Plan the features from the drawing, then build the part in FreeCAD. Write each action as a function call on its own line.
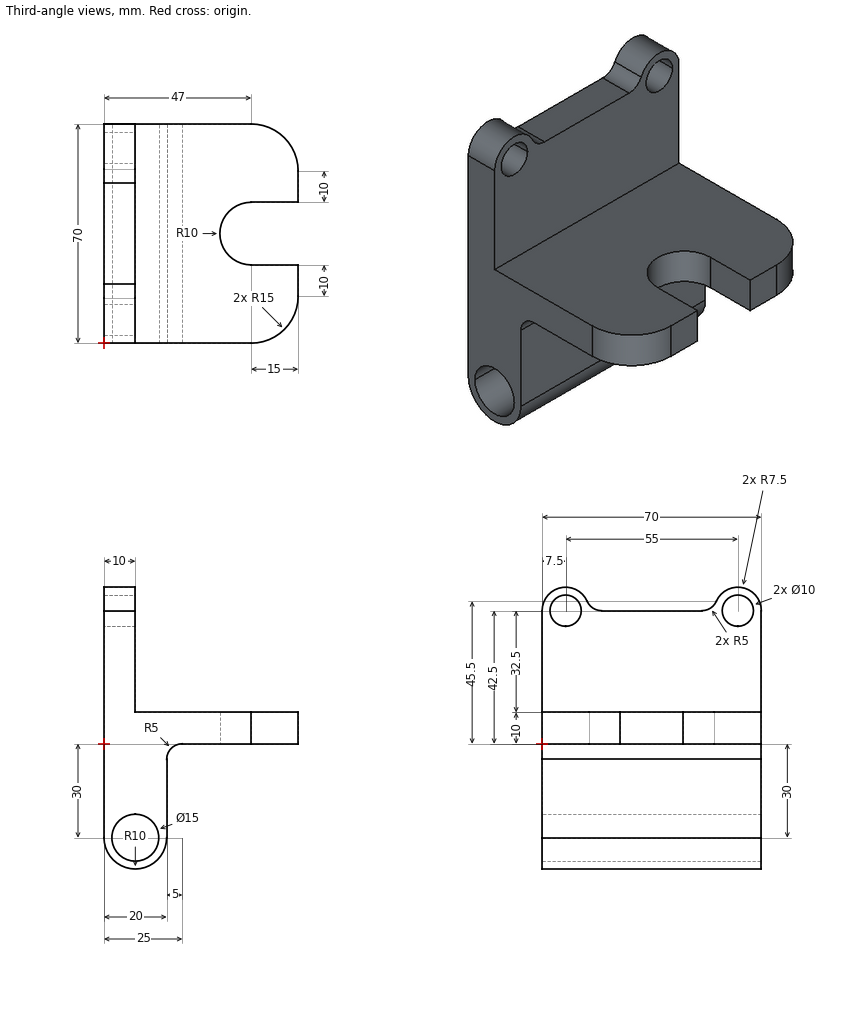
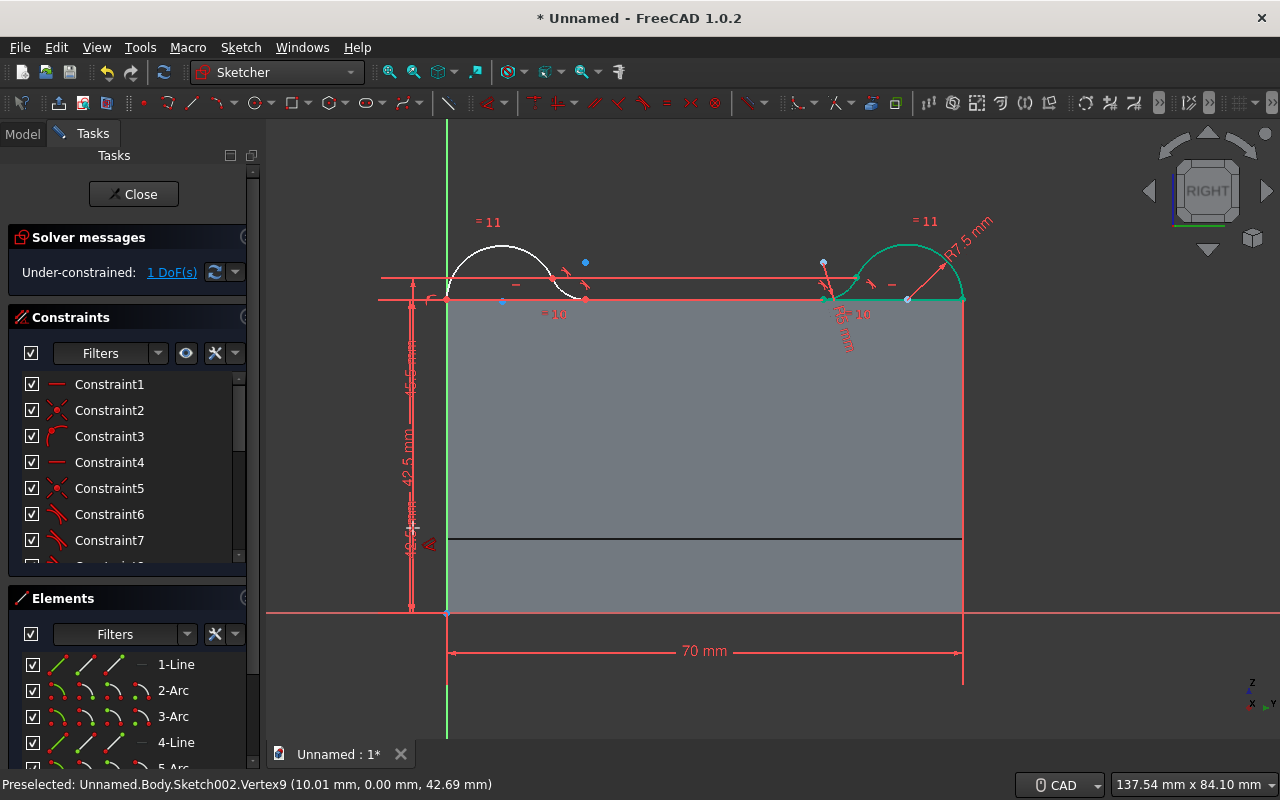
click(552, 278)
click(413, 329)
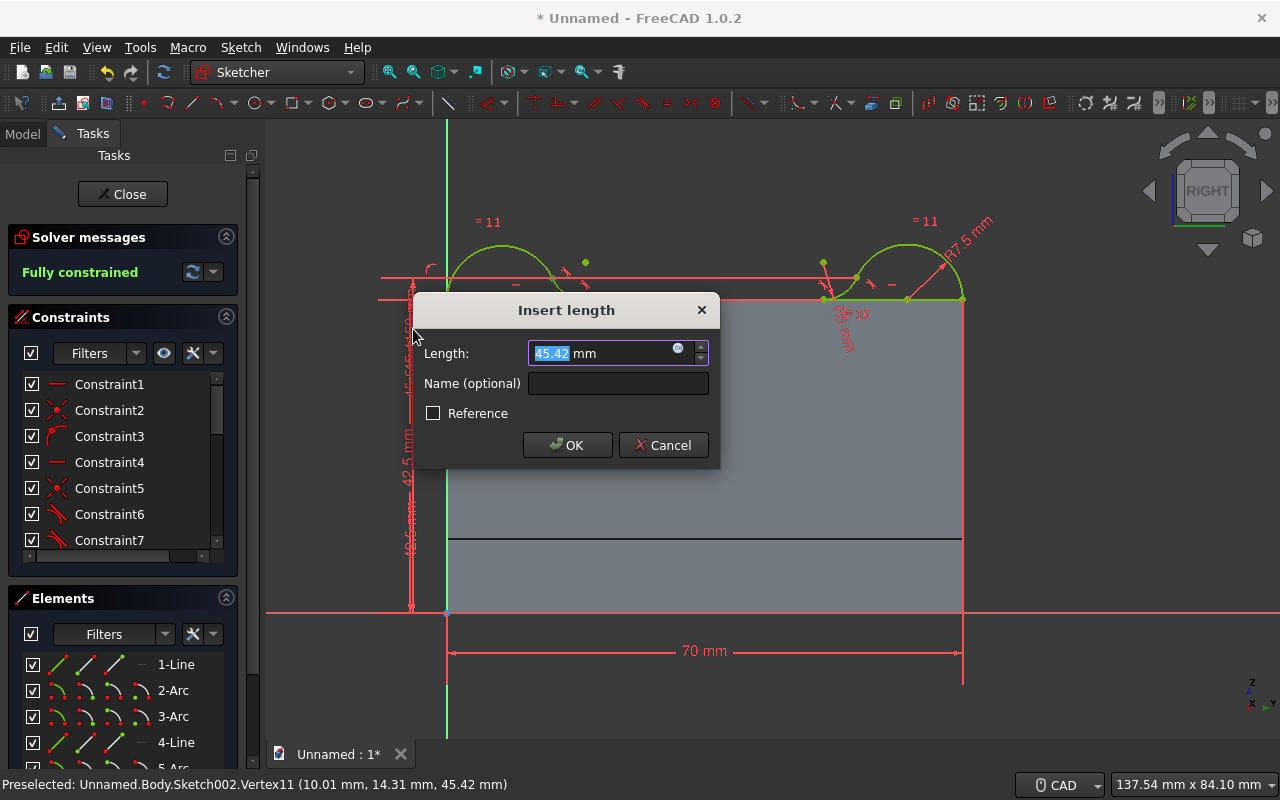
text(45.5)
key(Return)
key(Escape)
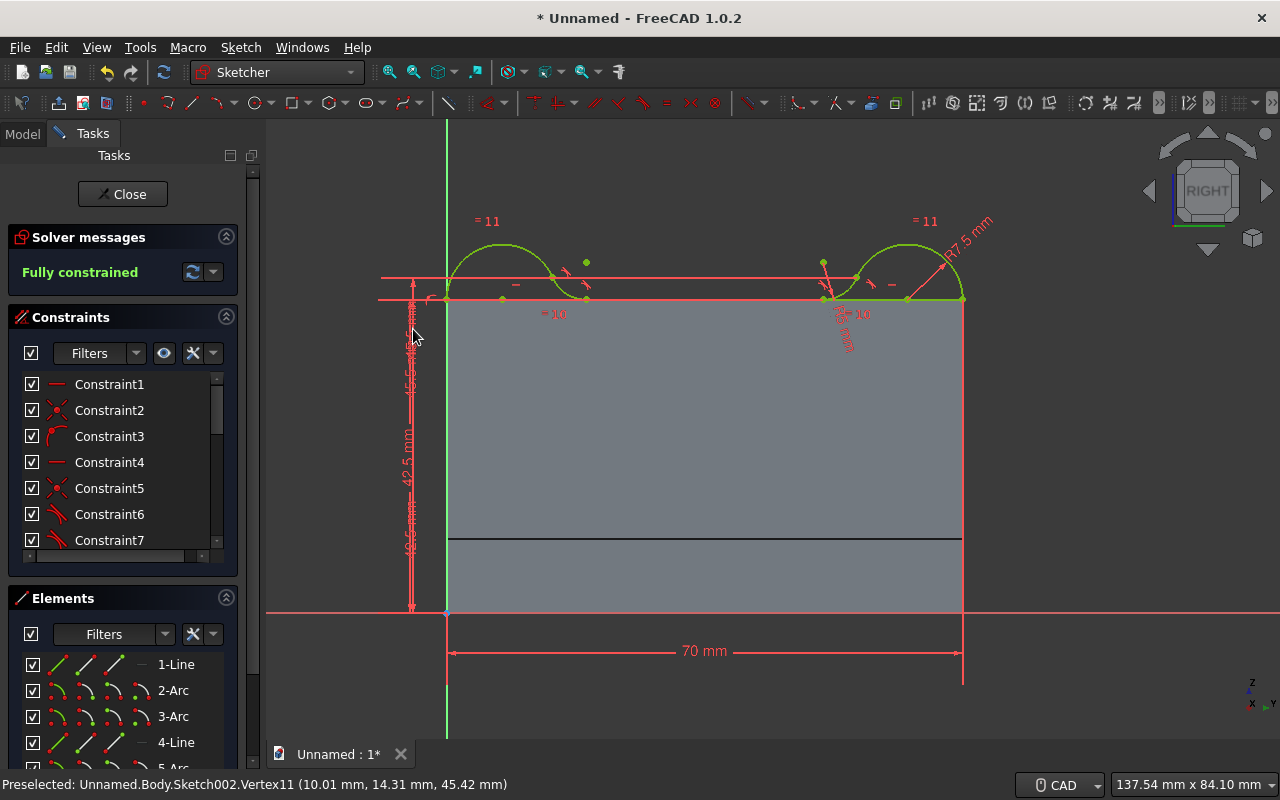
click(123, 194)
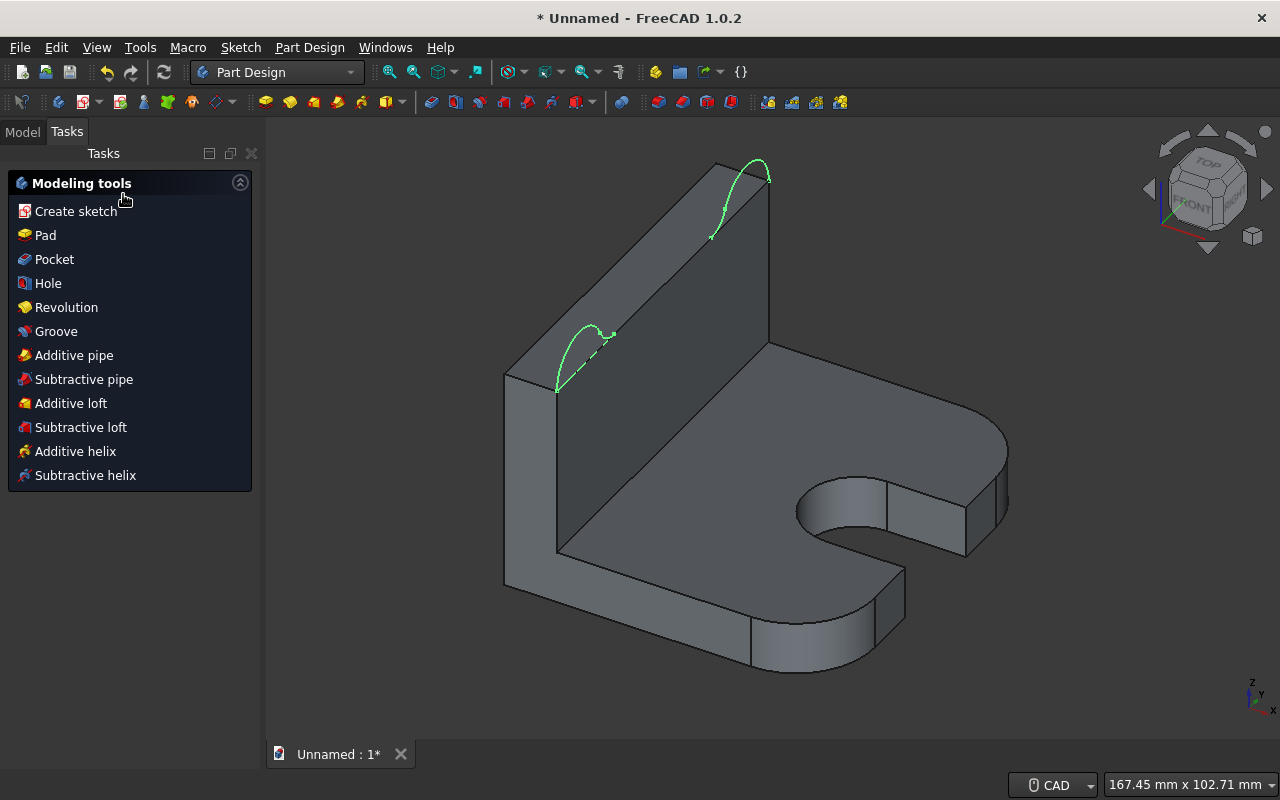
click(266, 102)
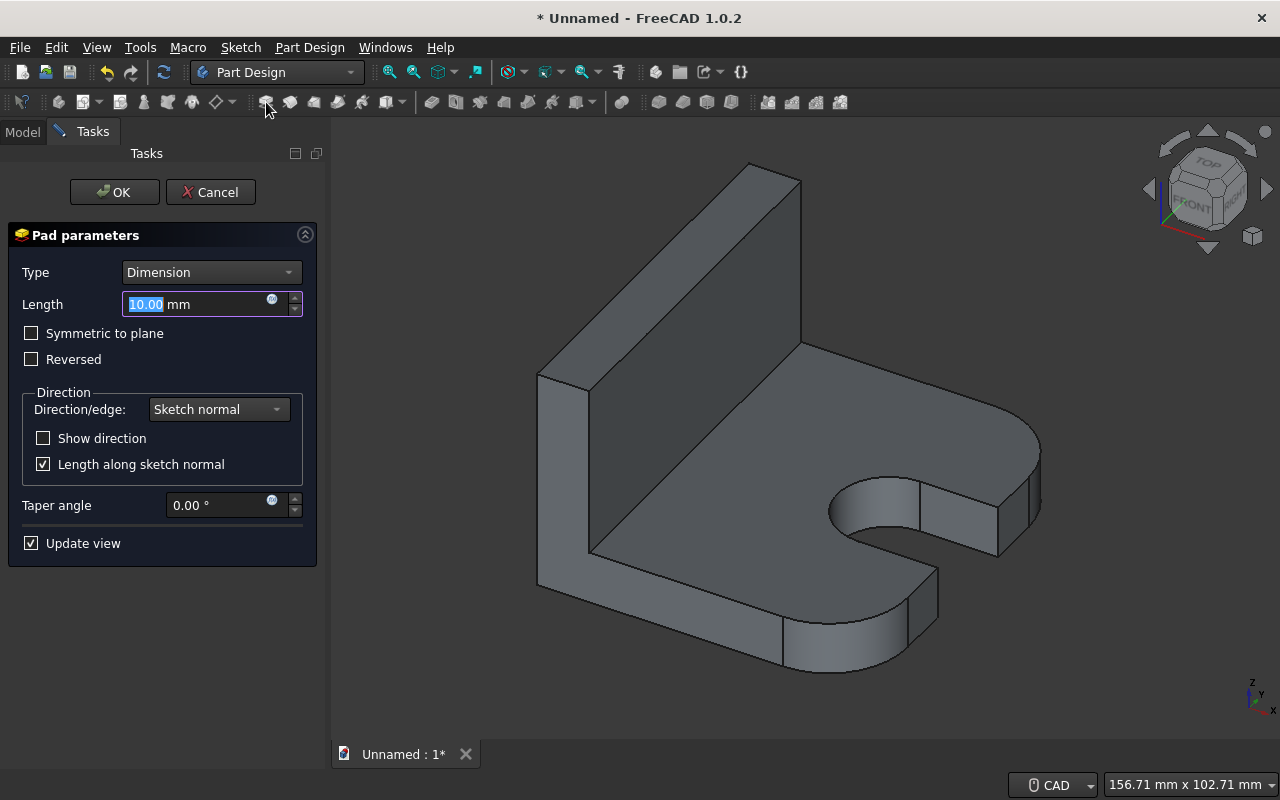
text(10)
key(Tab)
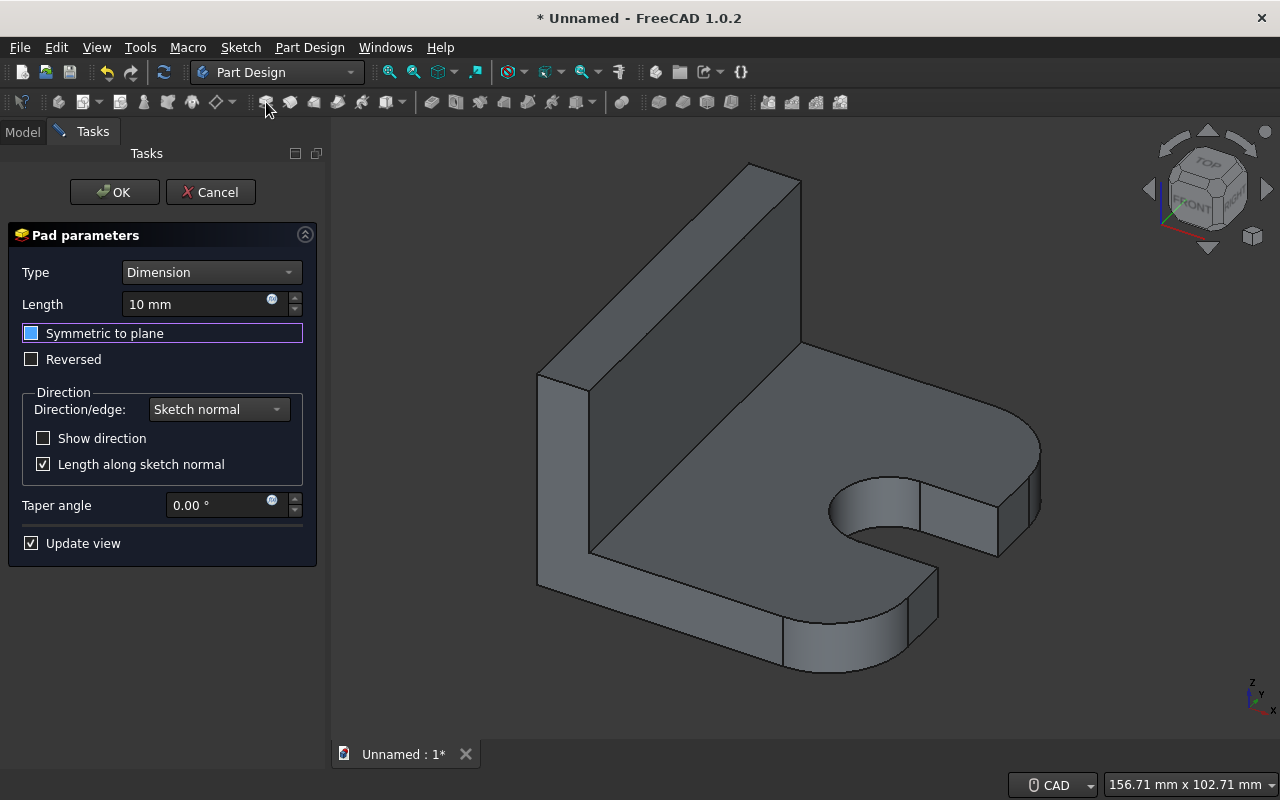
click(30, 359)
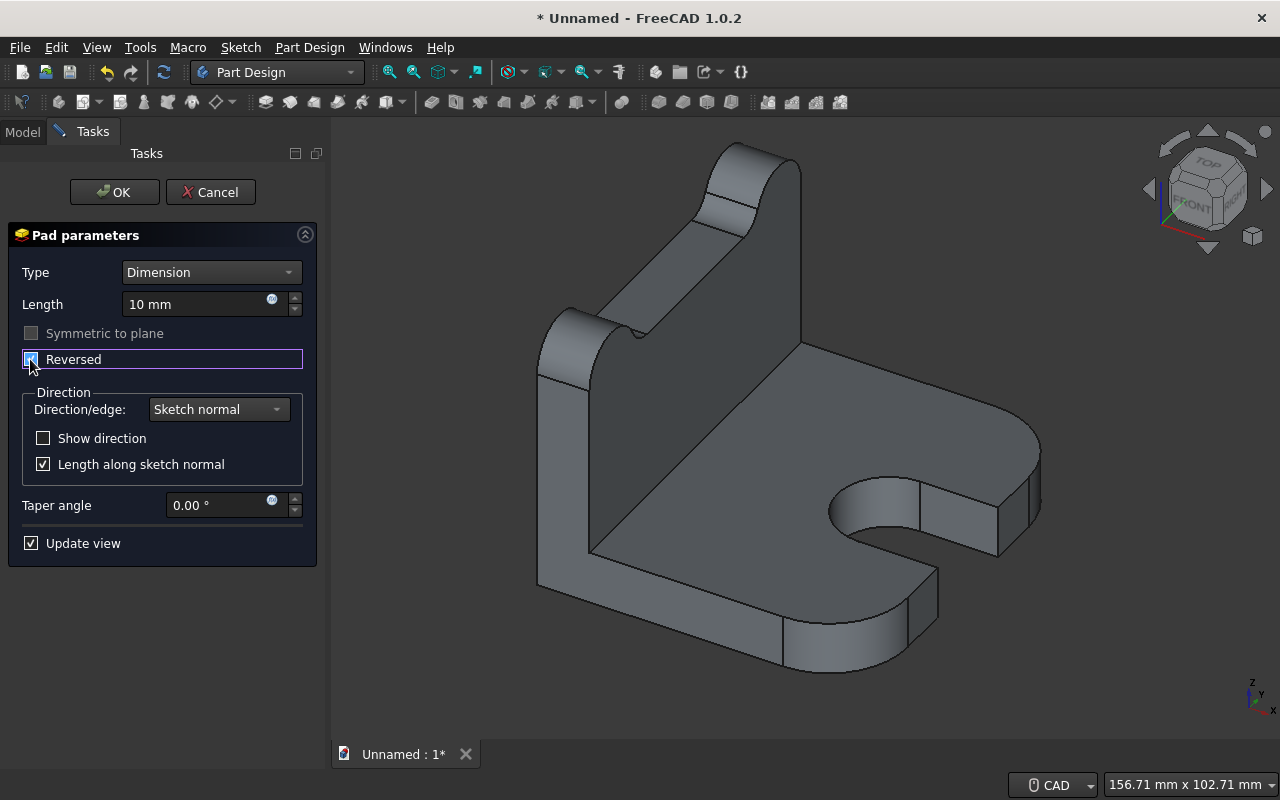
click(115, 192)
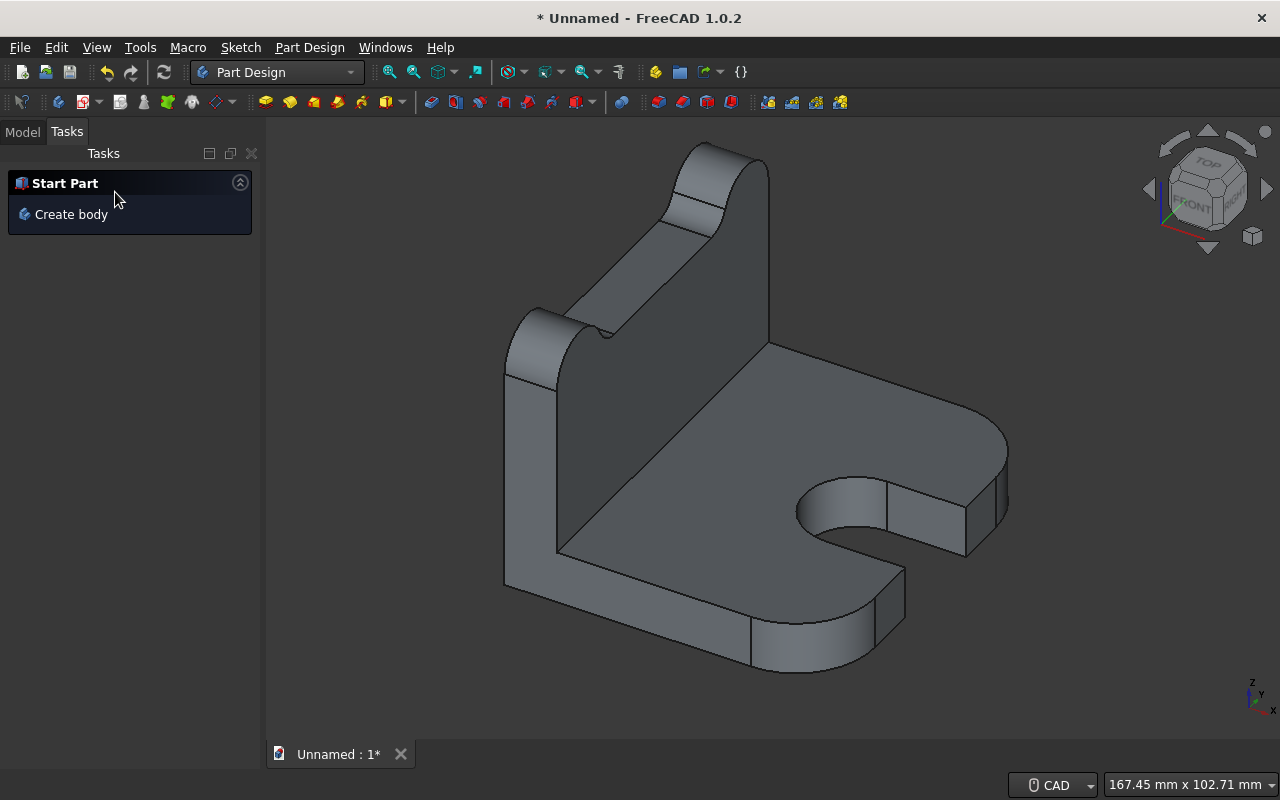
click(723, 315)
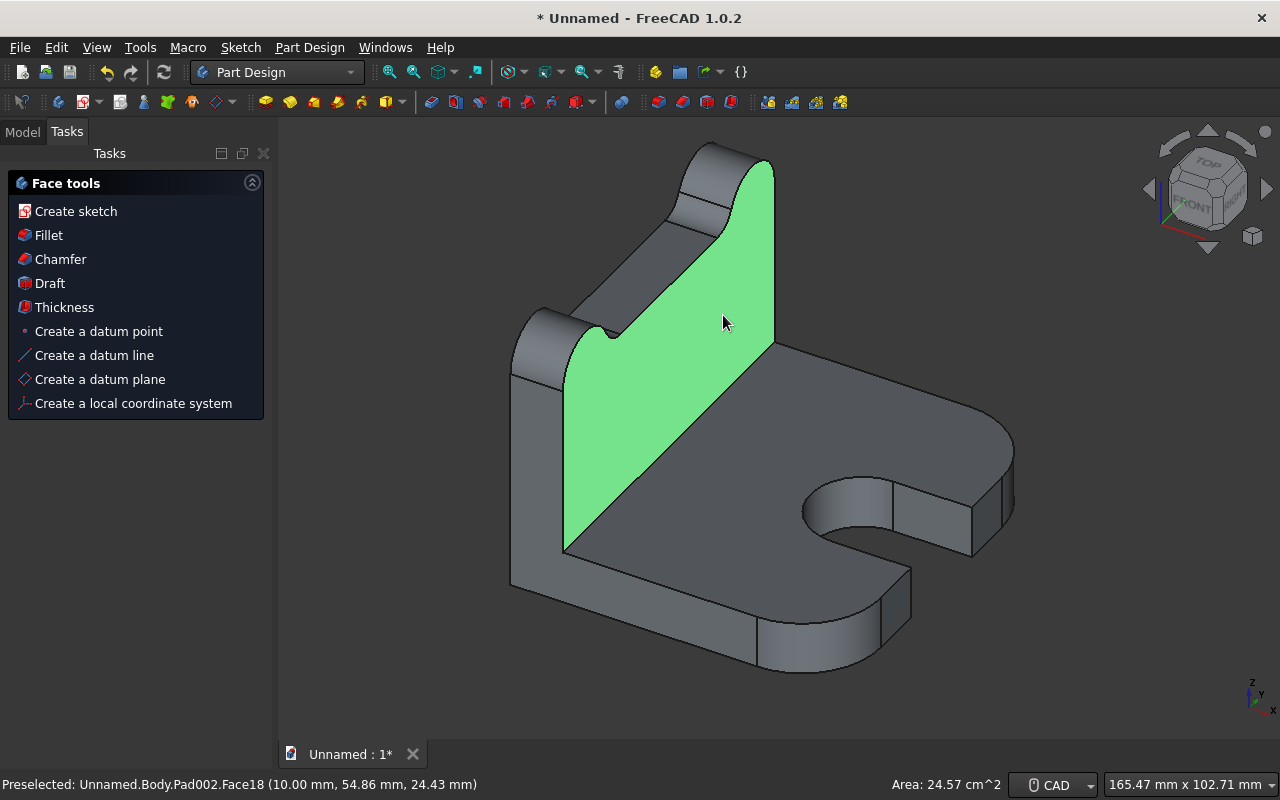
click(84, 102)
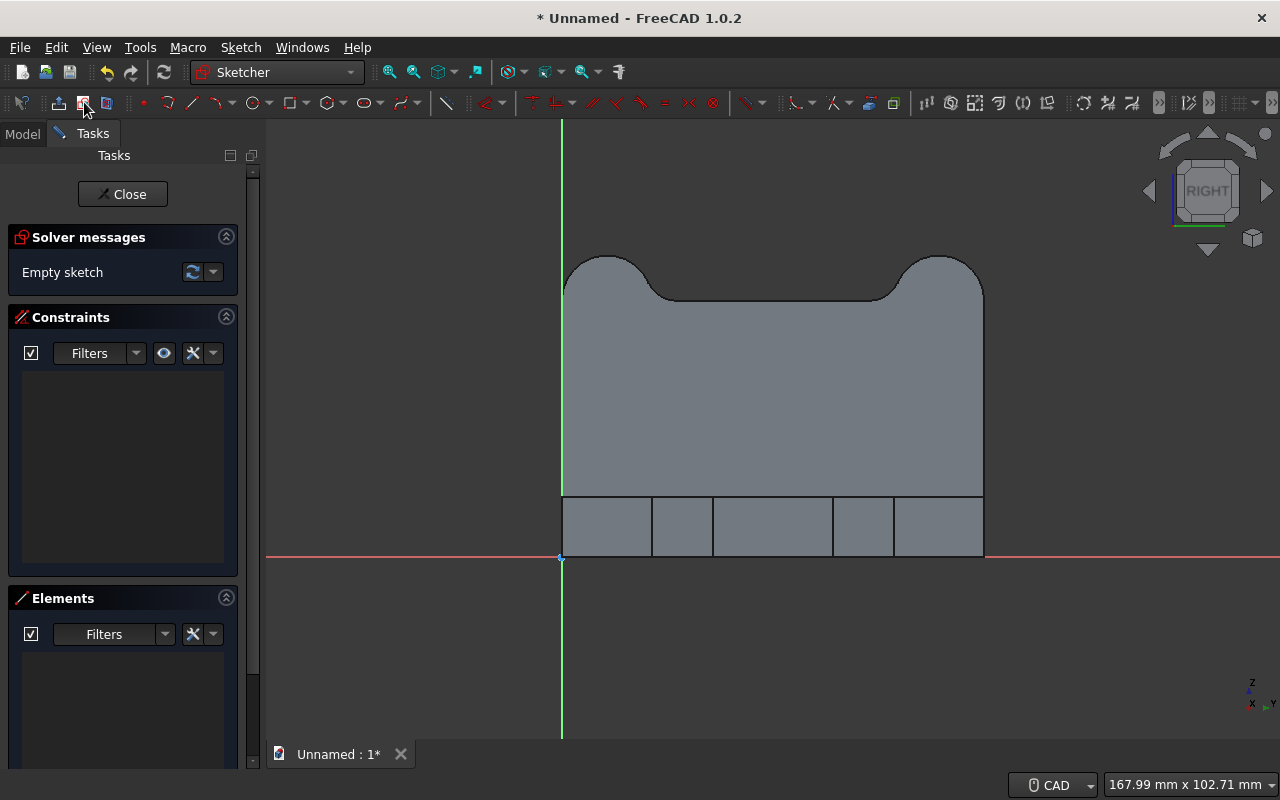
scroll(889, 383, up, 2)